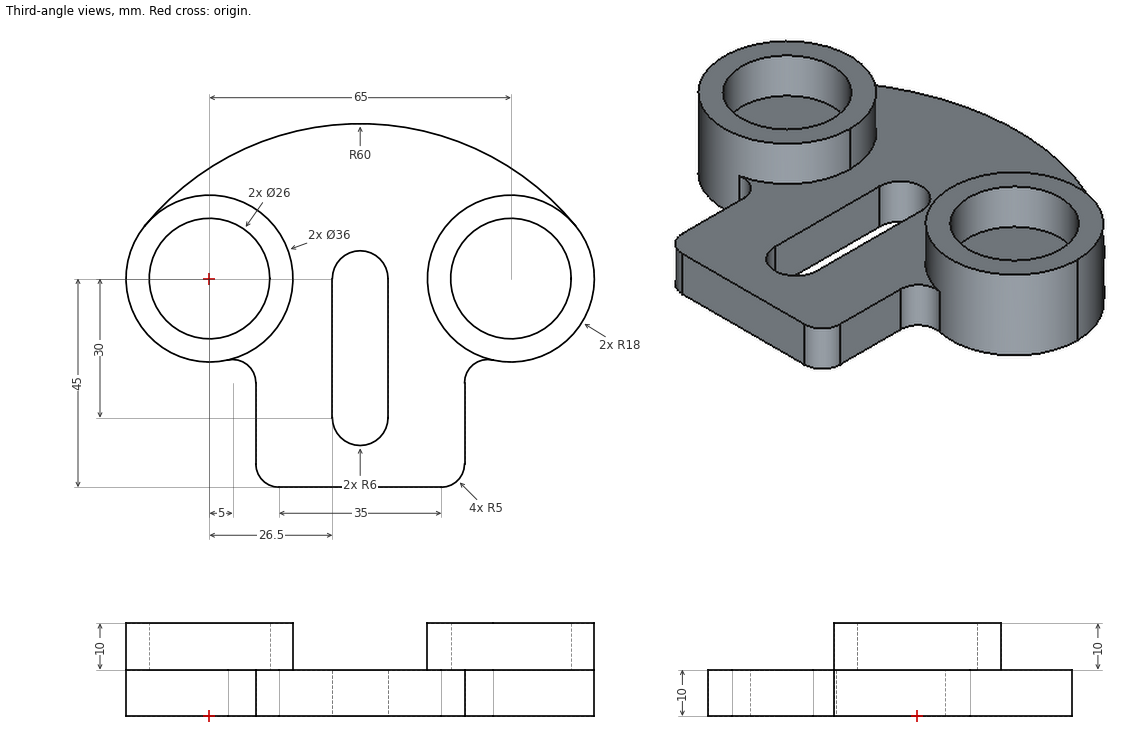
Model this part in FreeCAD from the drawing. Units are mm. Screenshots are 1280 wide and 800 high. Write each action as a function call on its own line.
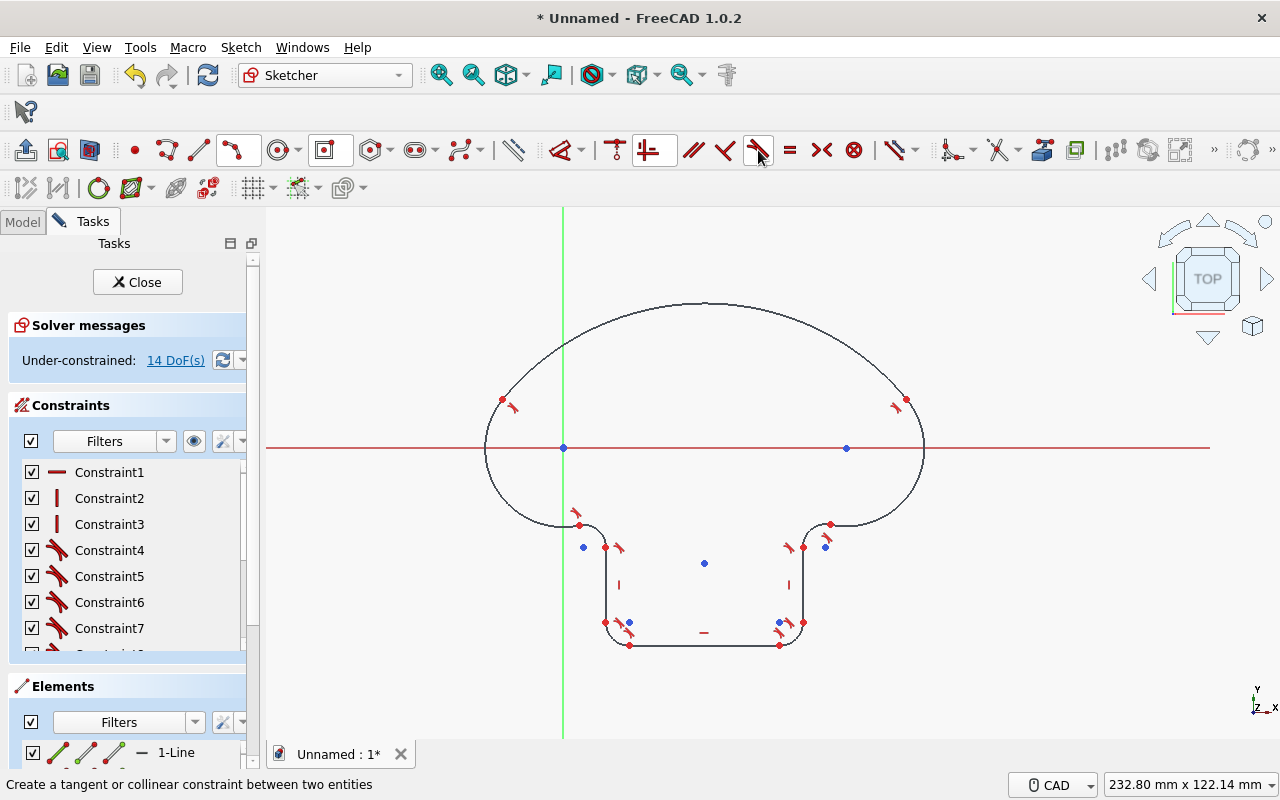
scroll(563, 448, up, 3)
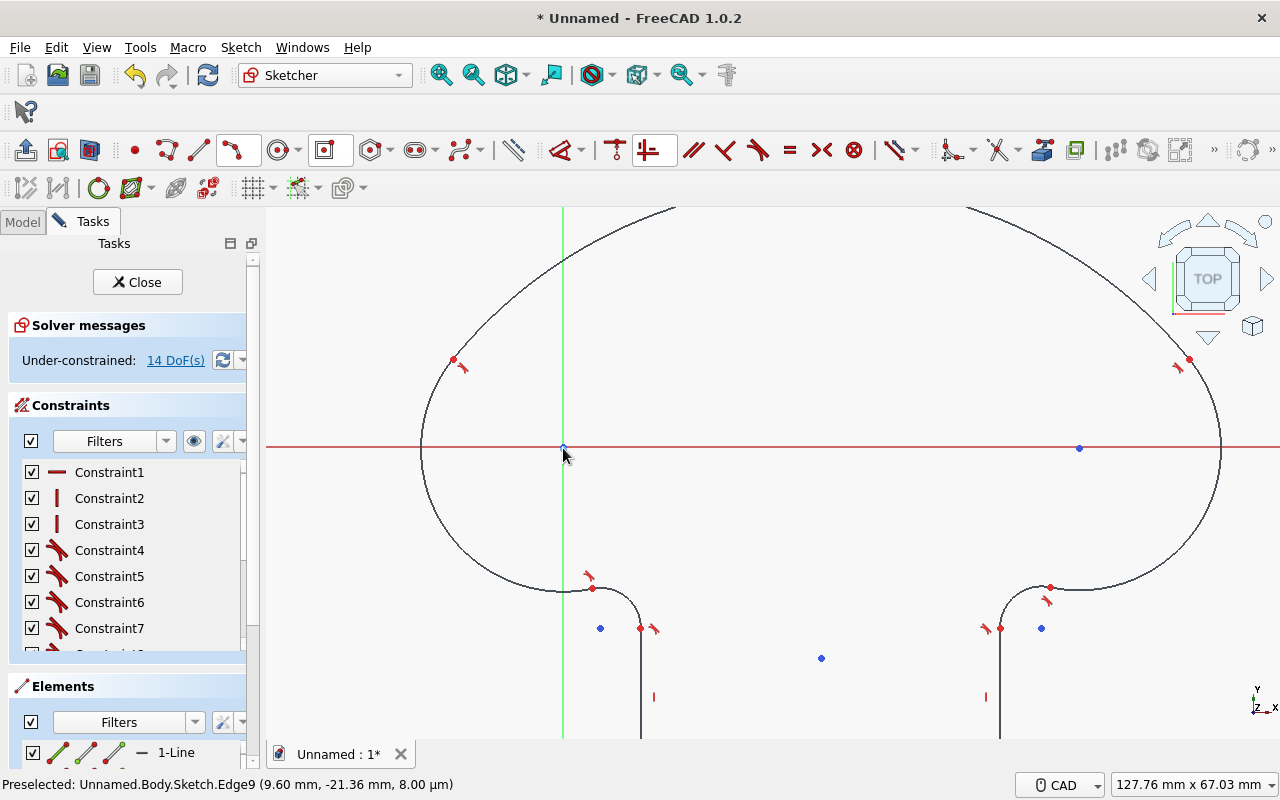
drag(553, 437, 574, 459)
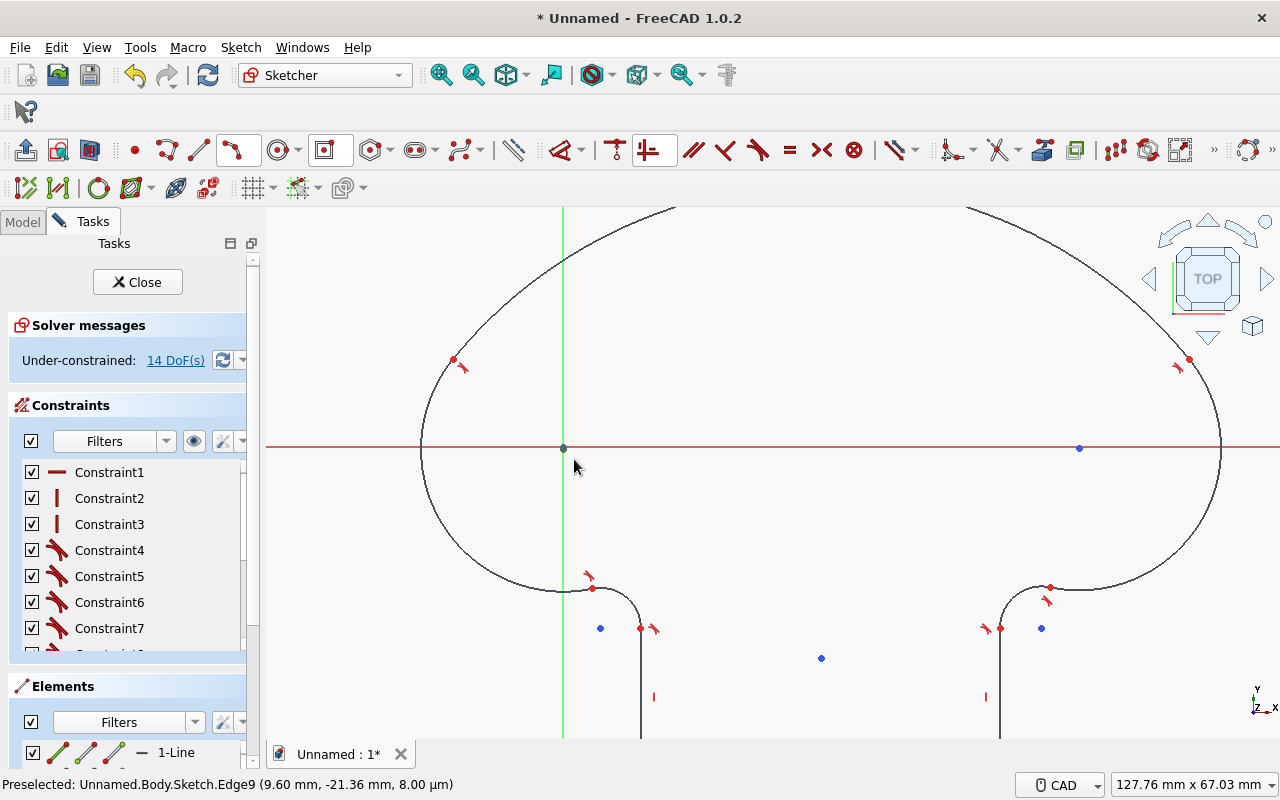
click(616, 150)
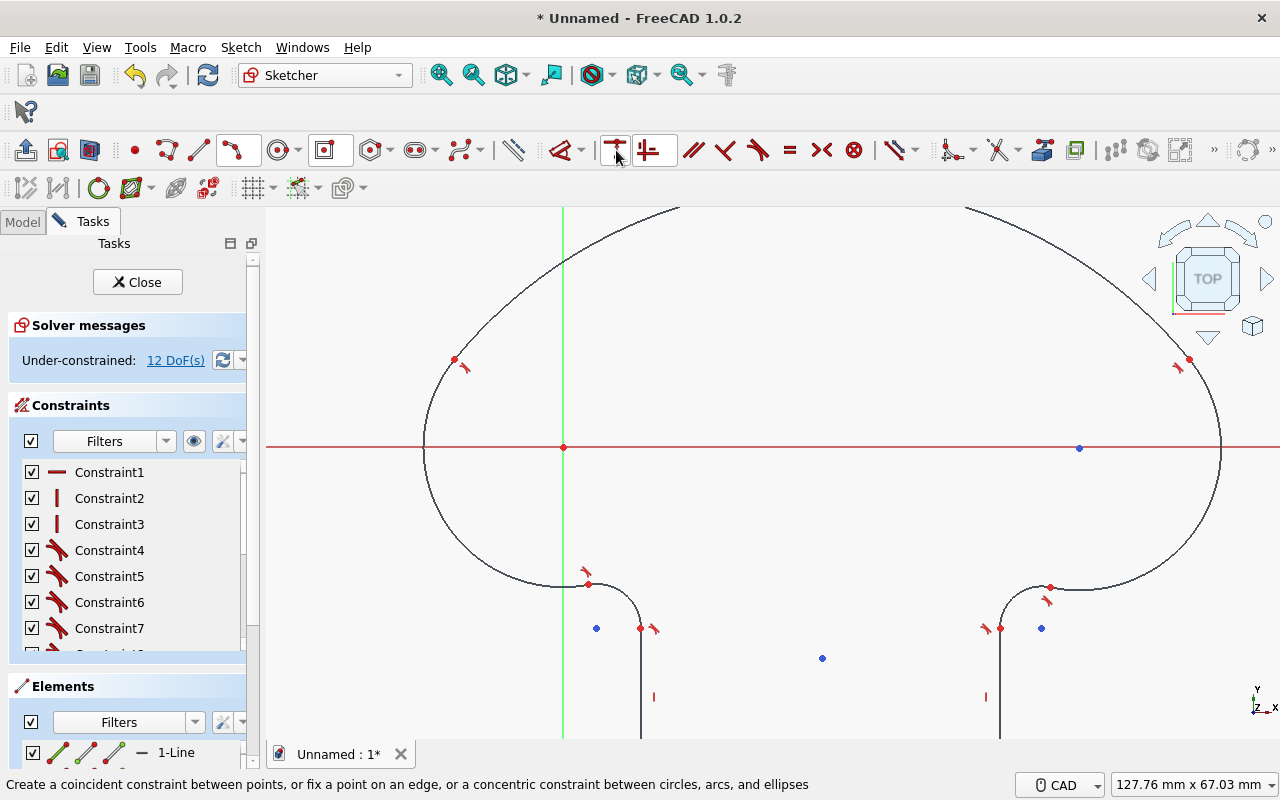
scroll(563, 448, down, 3)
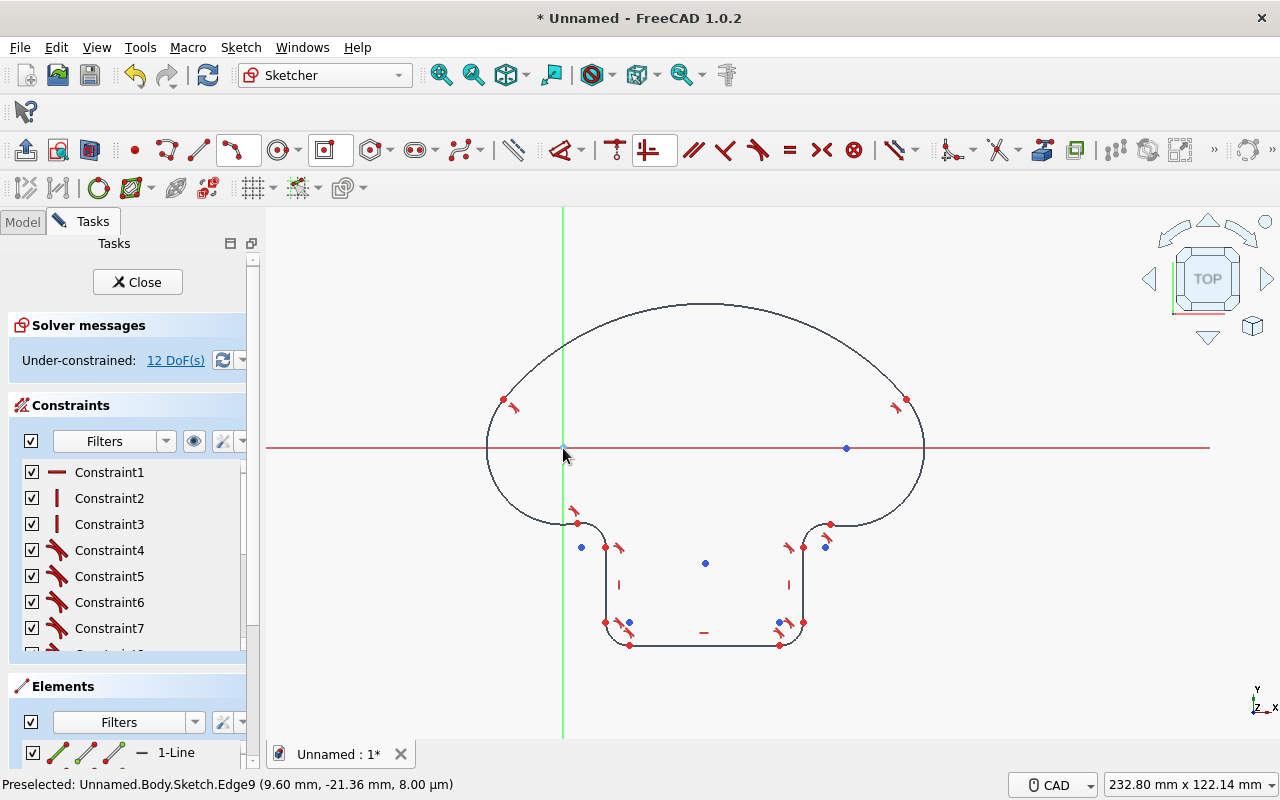
scroll(790, 643, up, 2)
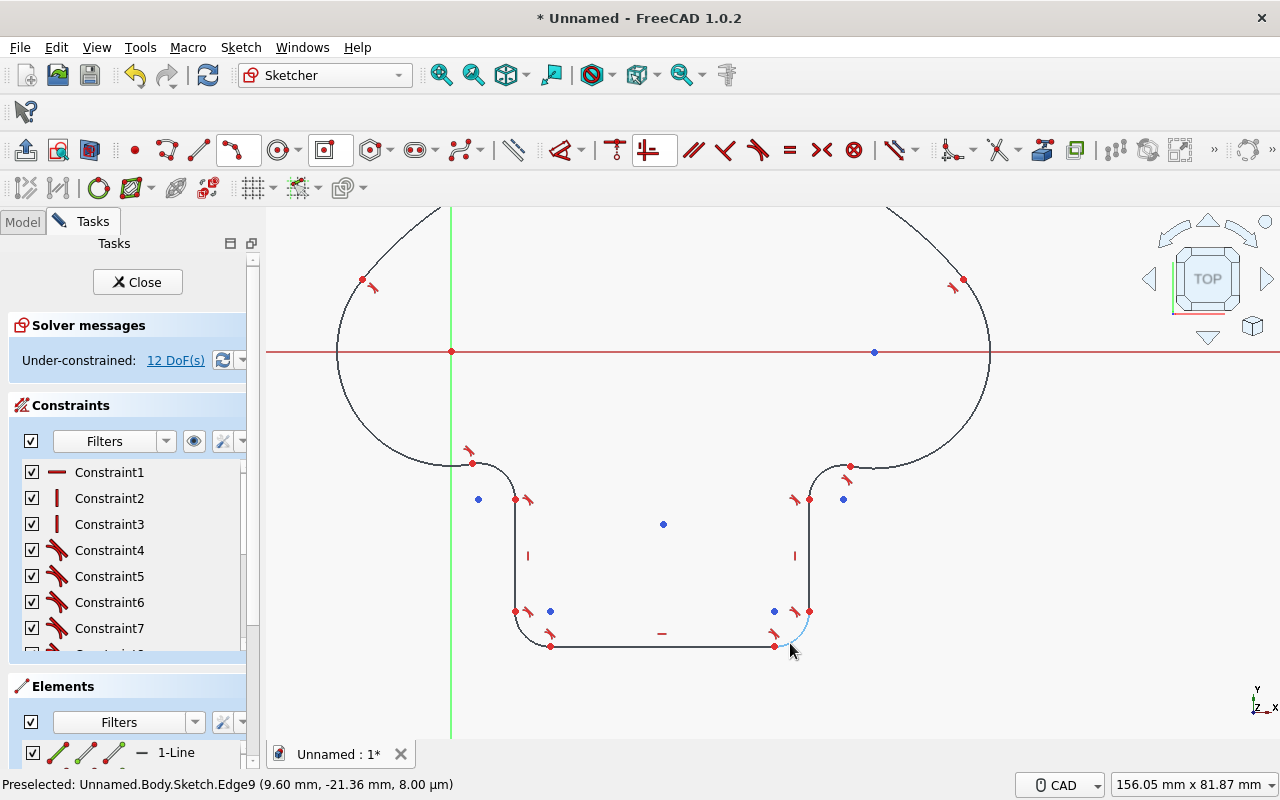
click(790, 643)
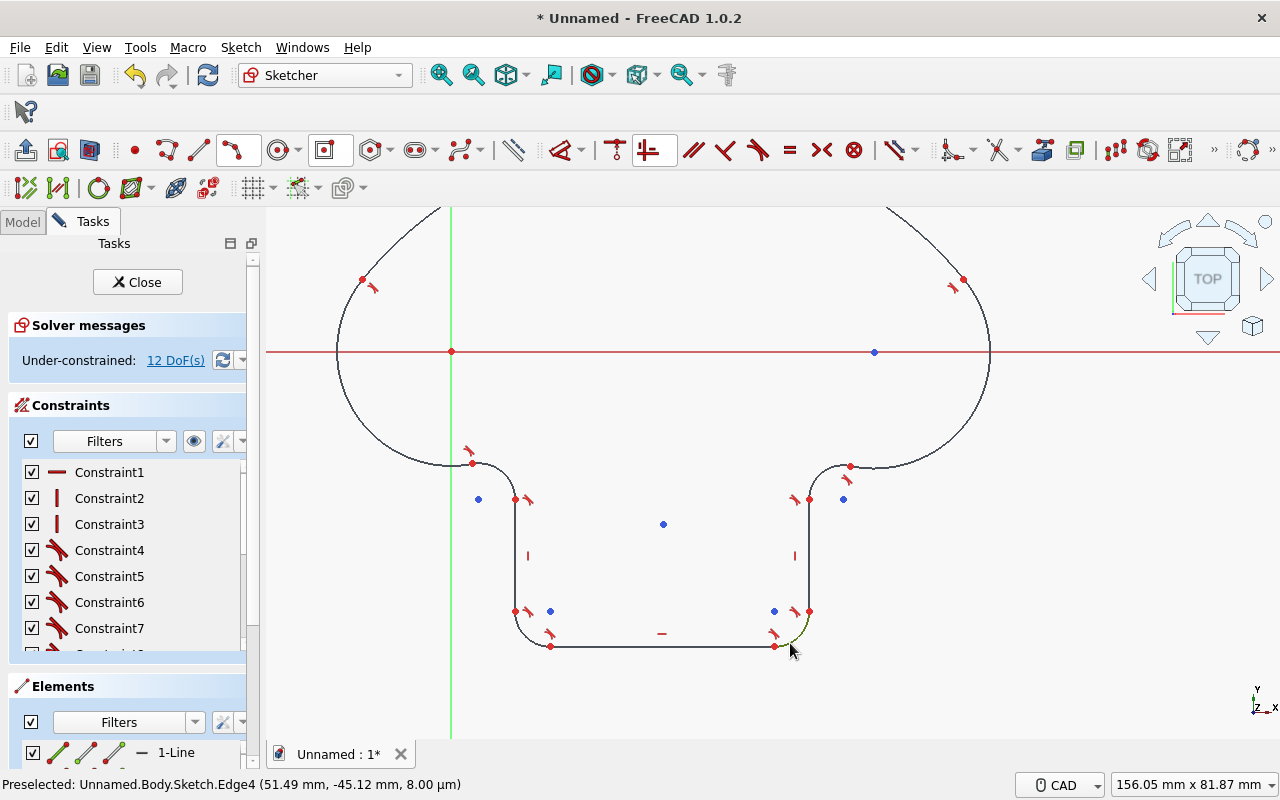
click(832, 467)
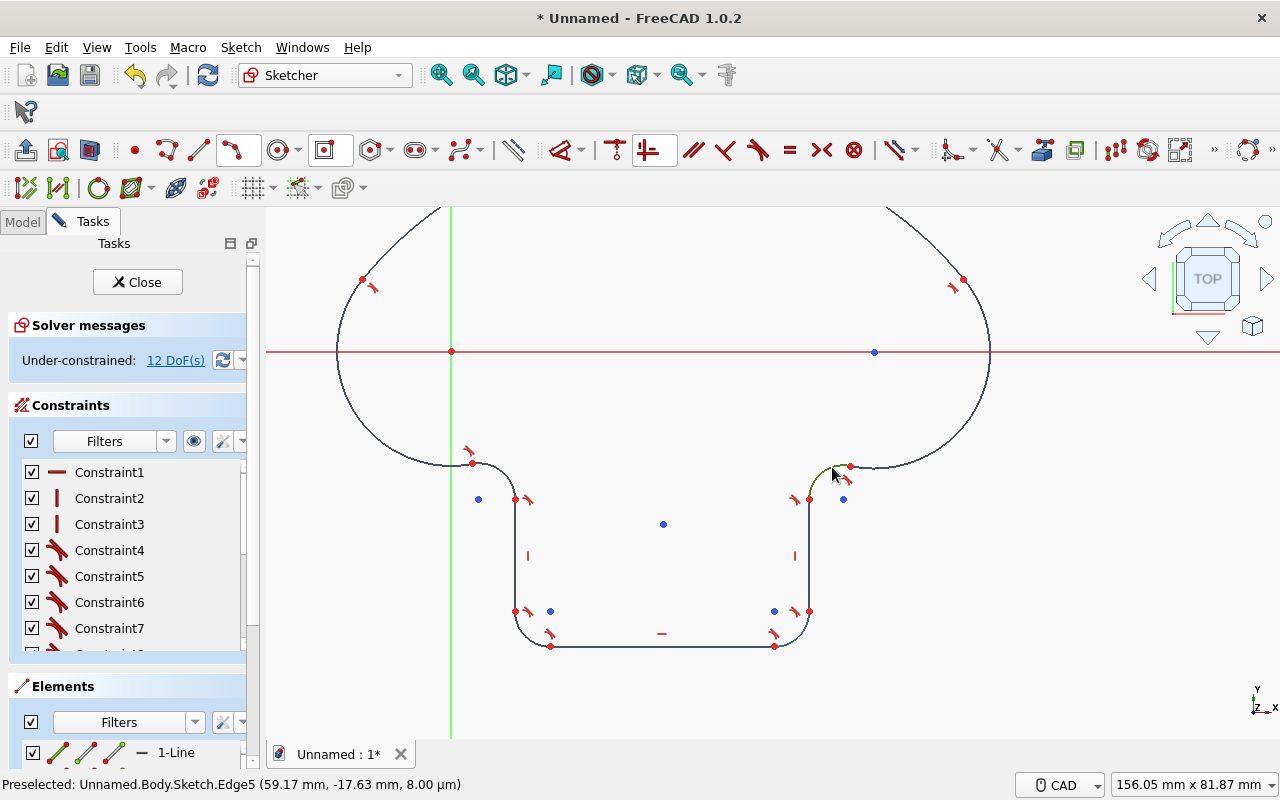
click(510, 481)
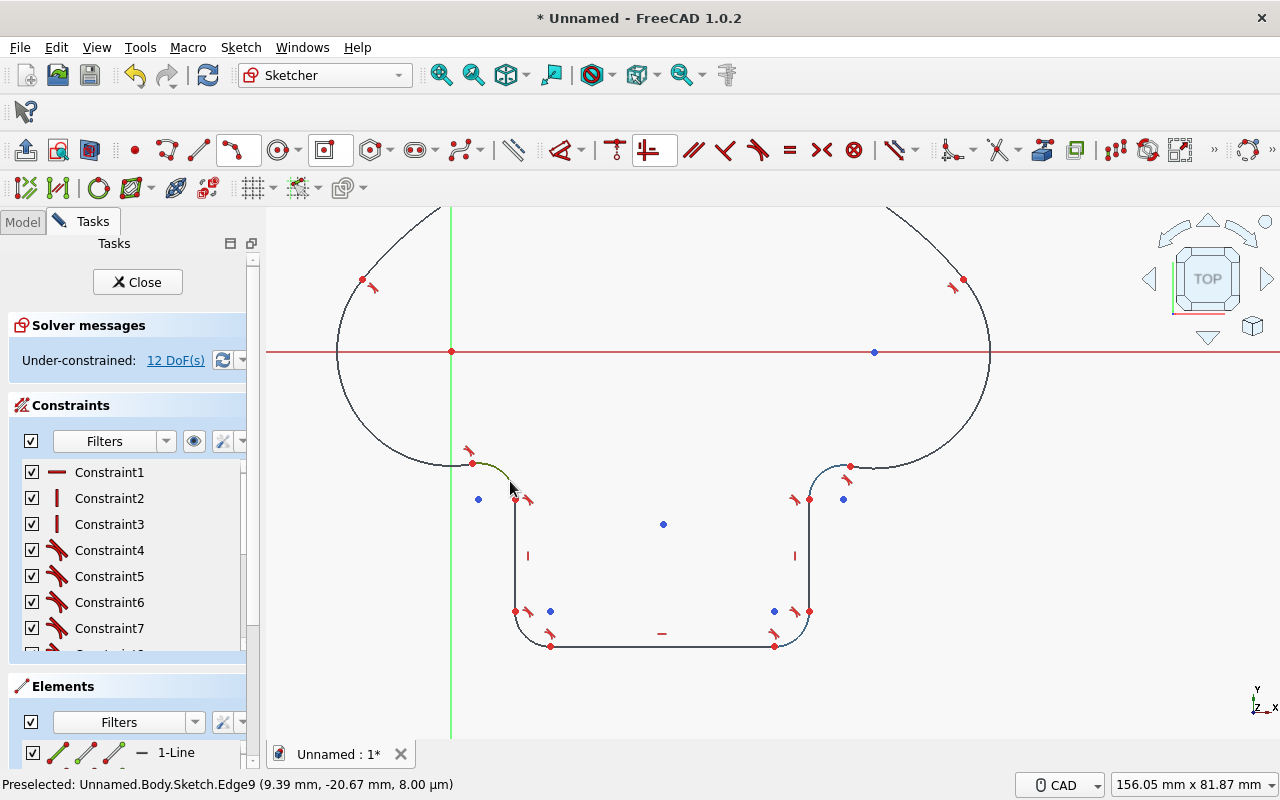
click(519, 627)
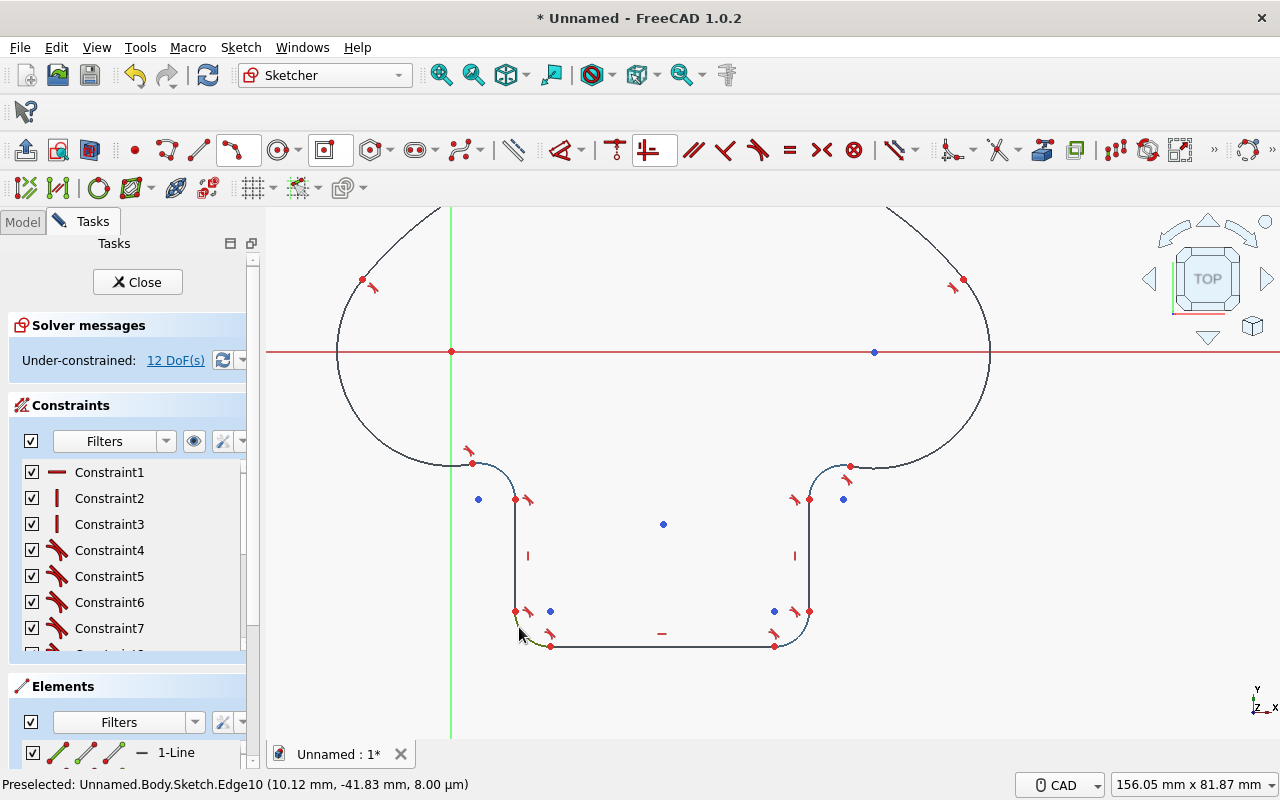
click(790, 150)